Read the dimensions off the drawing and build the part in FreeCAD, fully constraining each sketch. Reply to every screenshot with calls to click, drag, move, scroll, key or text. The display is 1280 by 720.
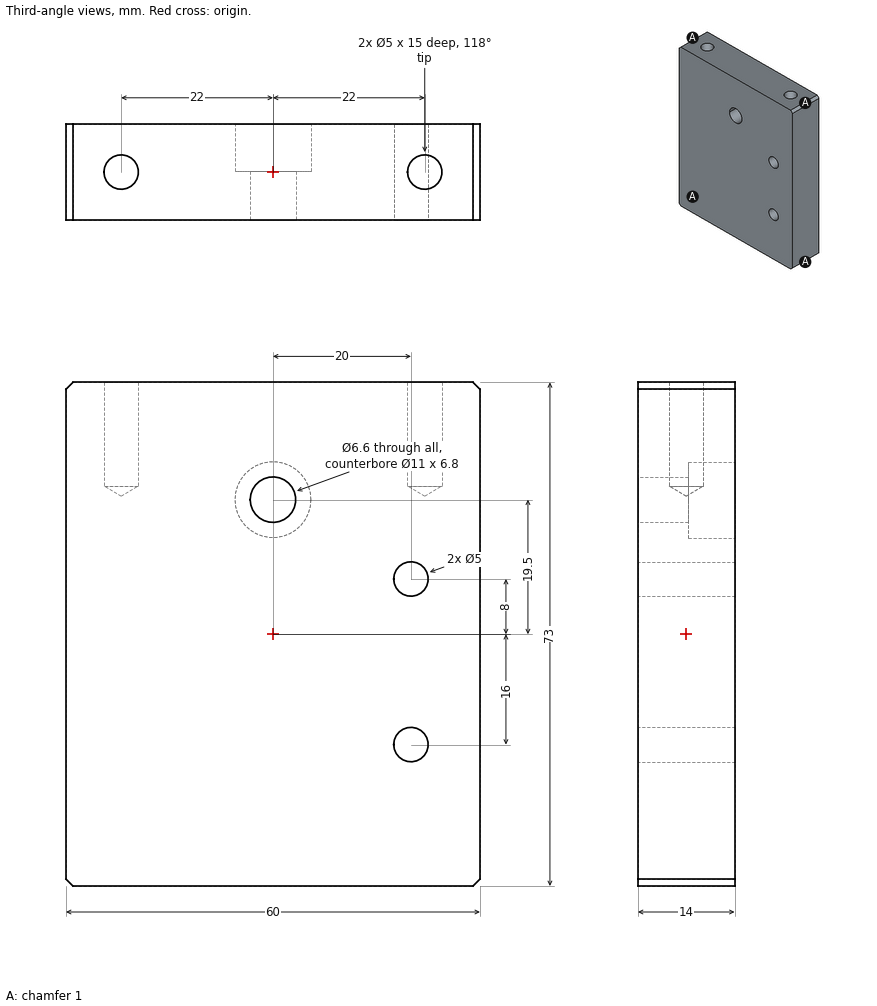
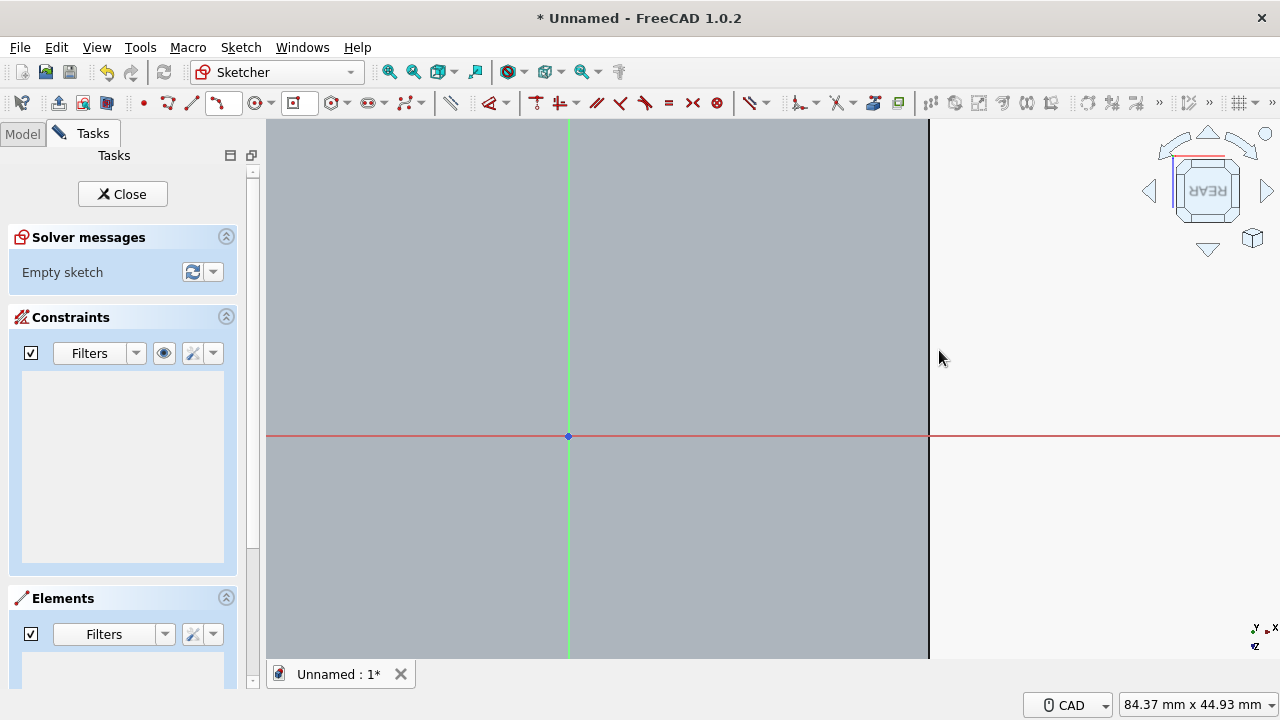
click(256, 104)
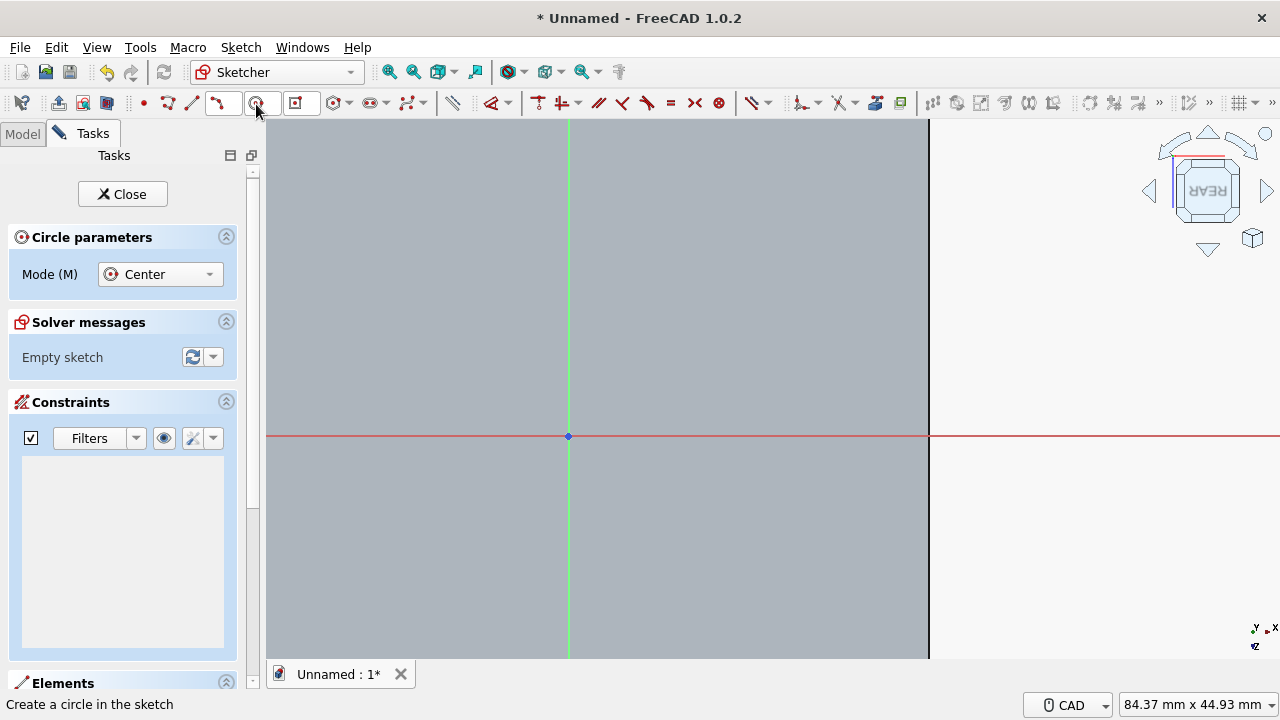
click(809, 532)
click(830, 511)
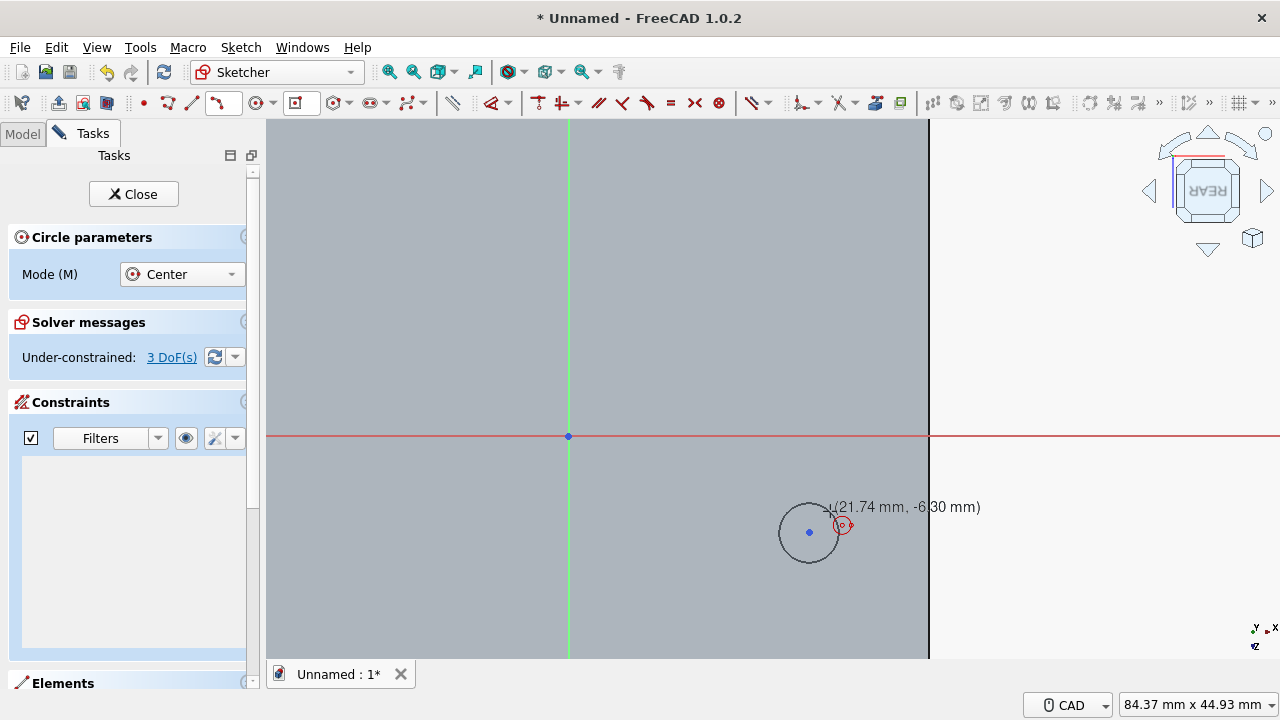
click(809, 244)
click(830, 223)
key(Escape)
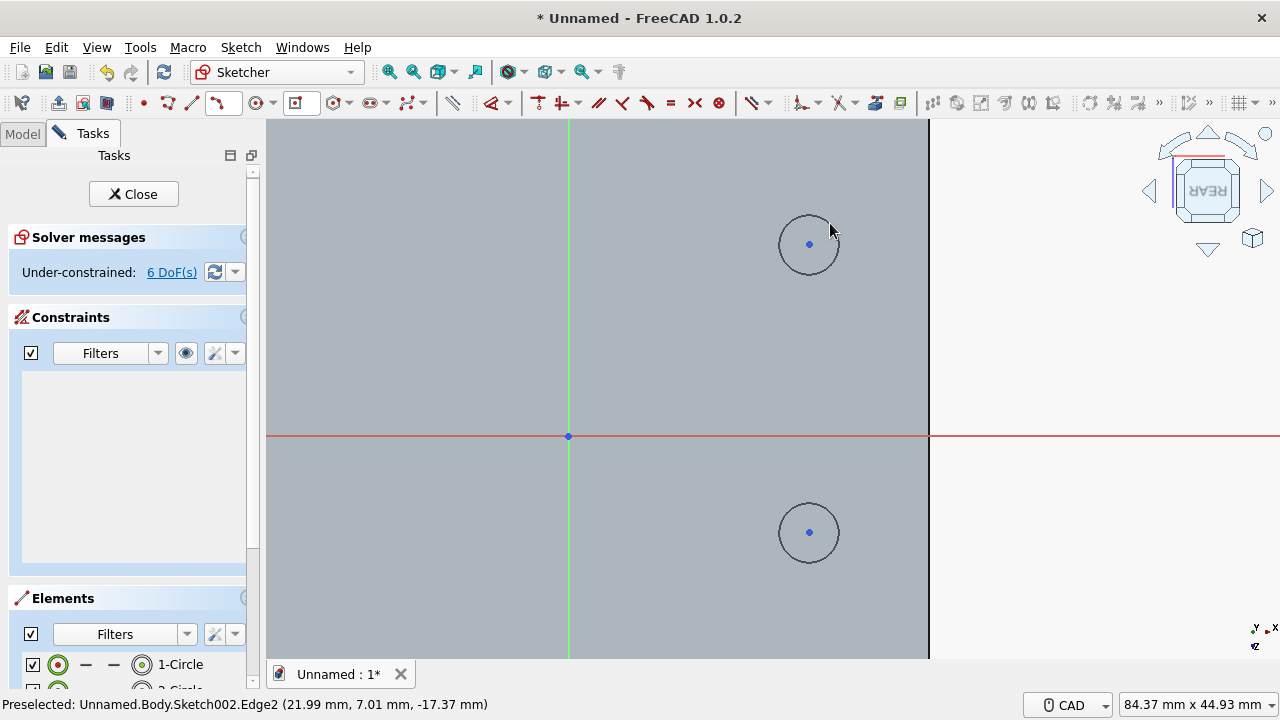
click(830, 512)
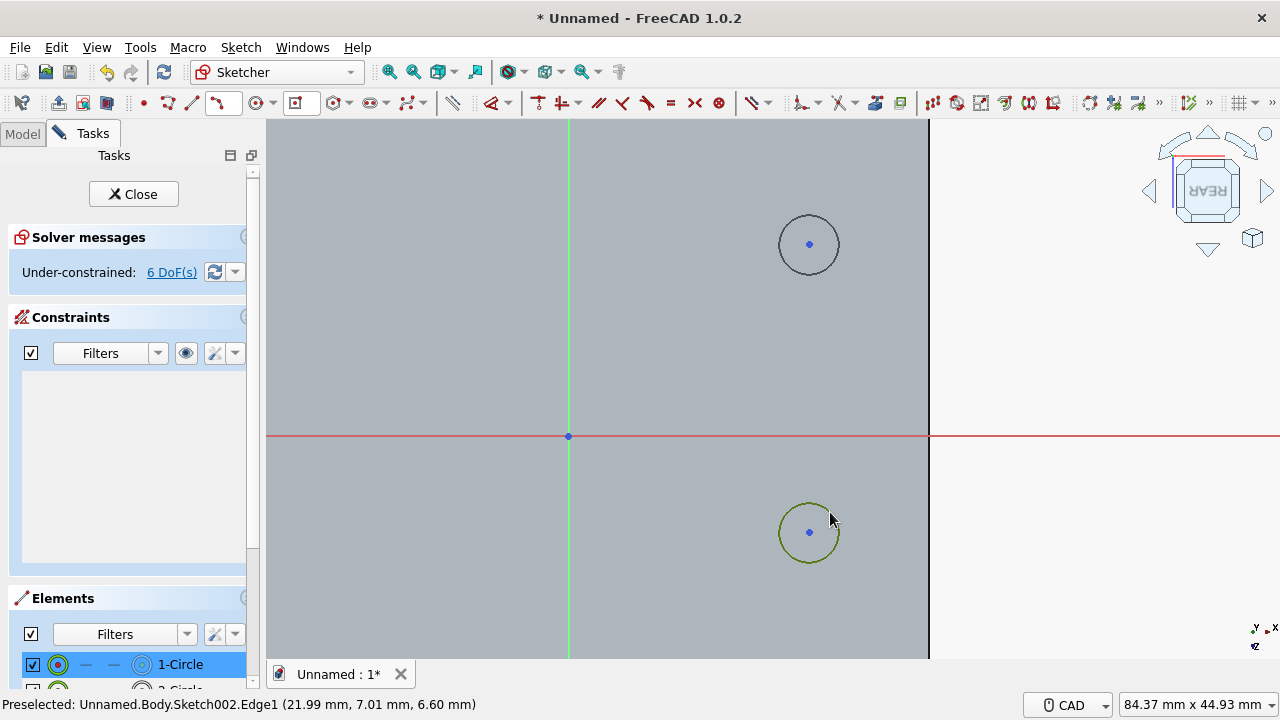
click(830, 224)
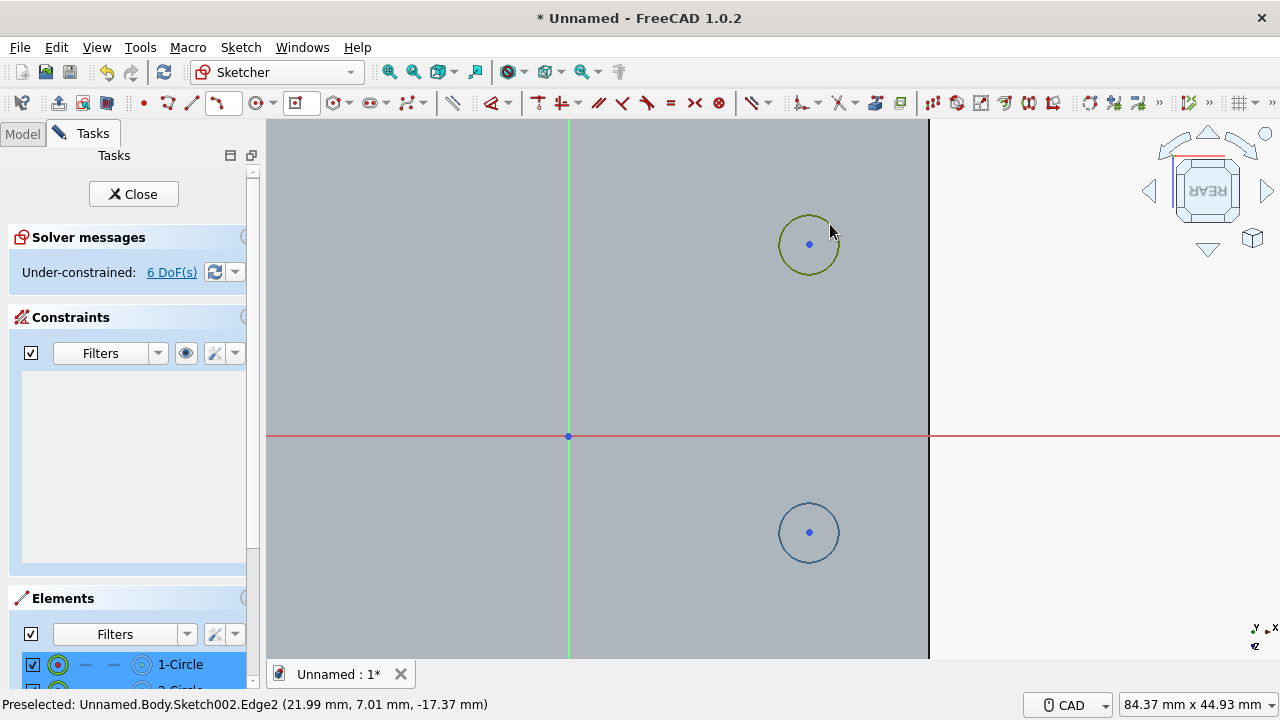
click(672, 104)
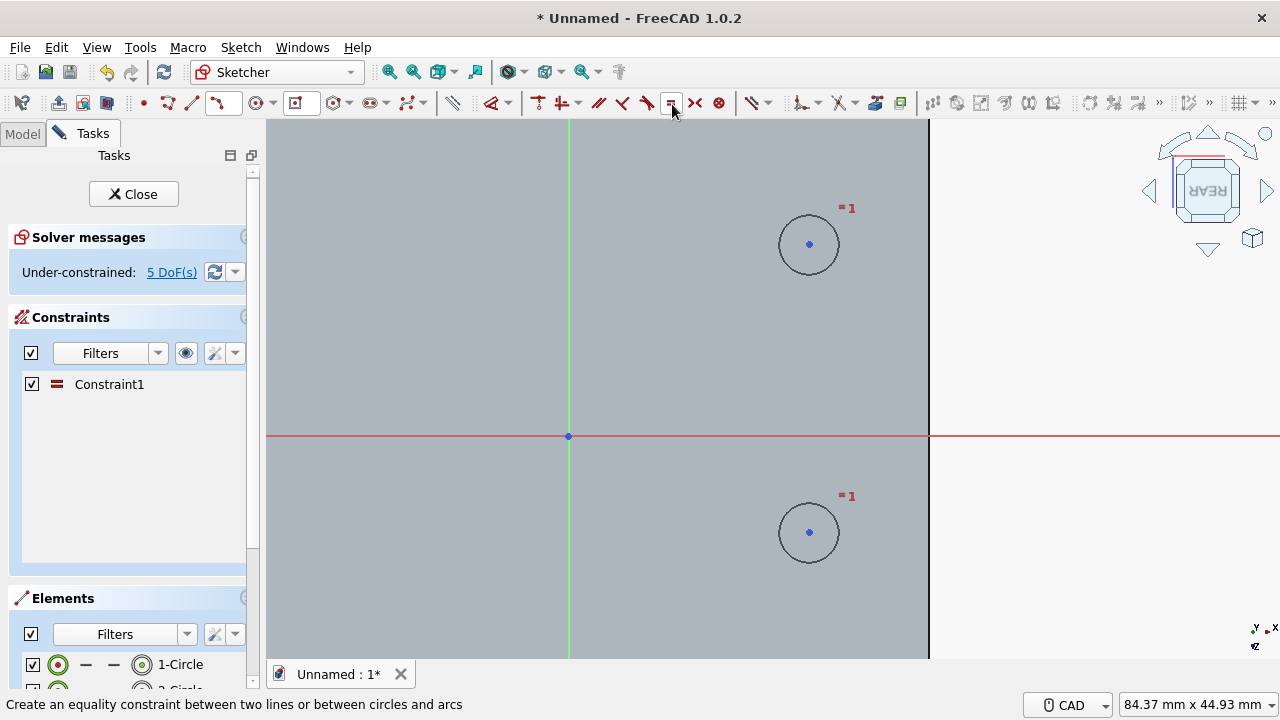
click(809, 533)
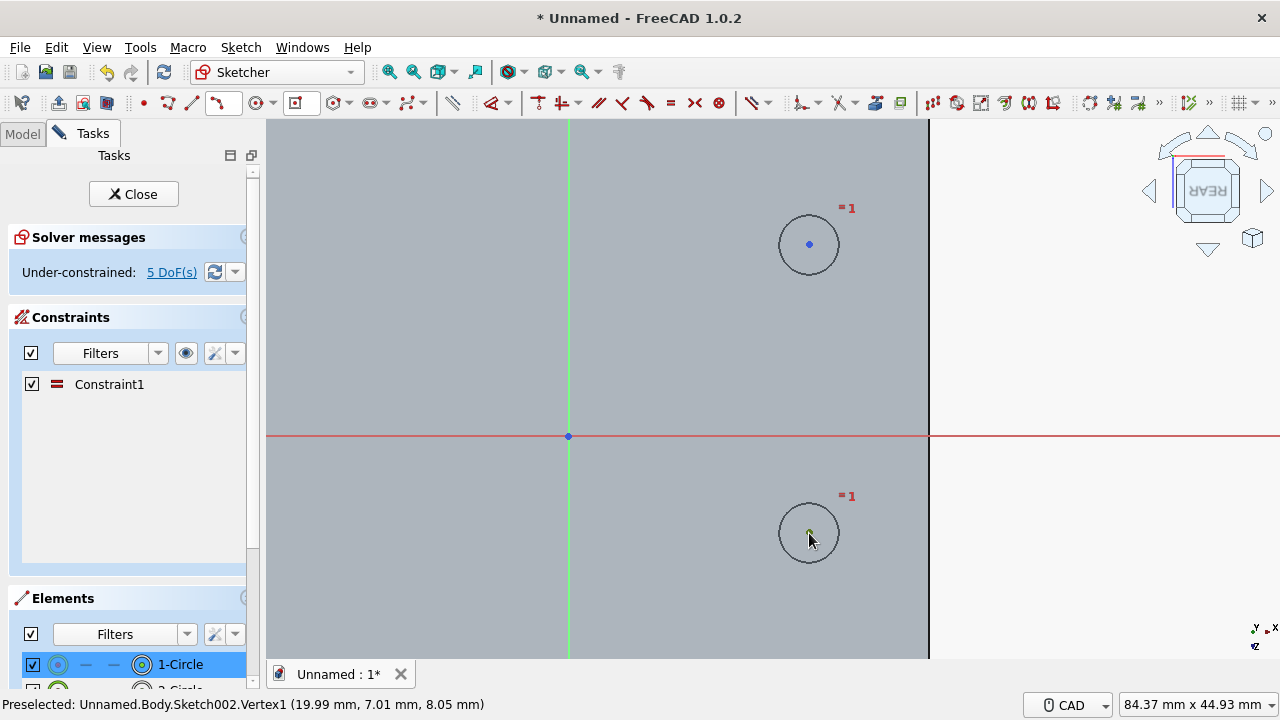
click(809, 245)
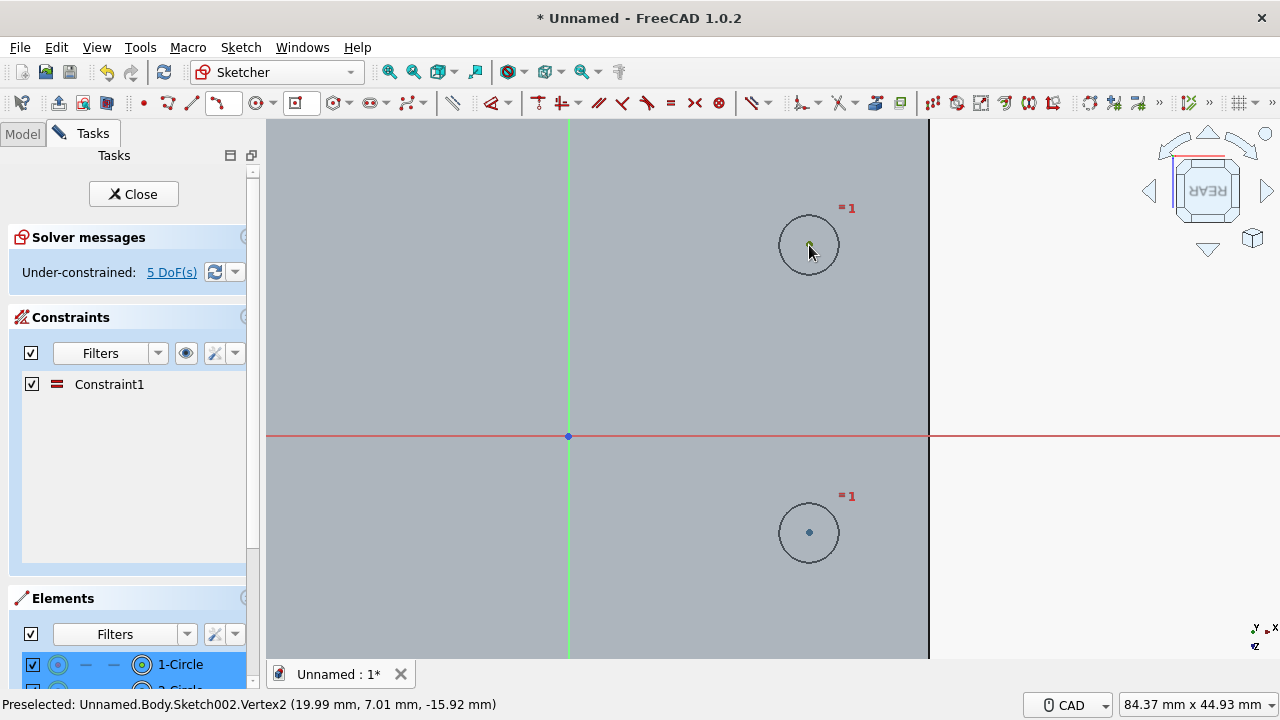
click(580, 104)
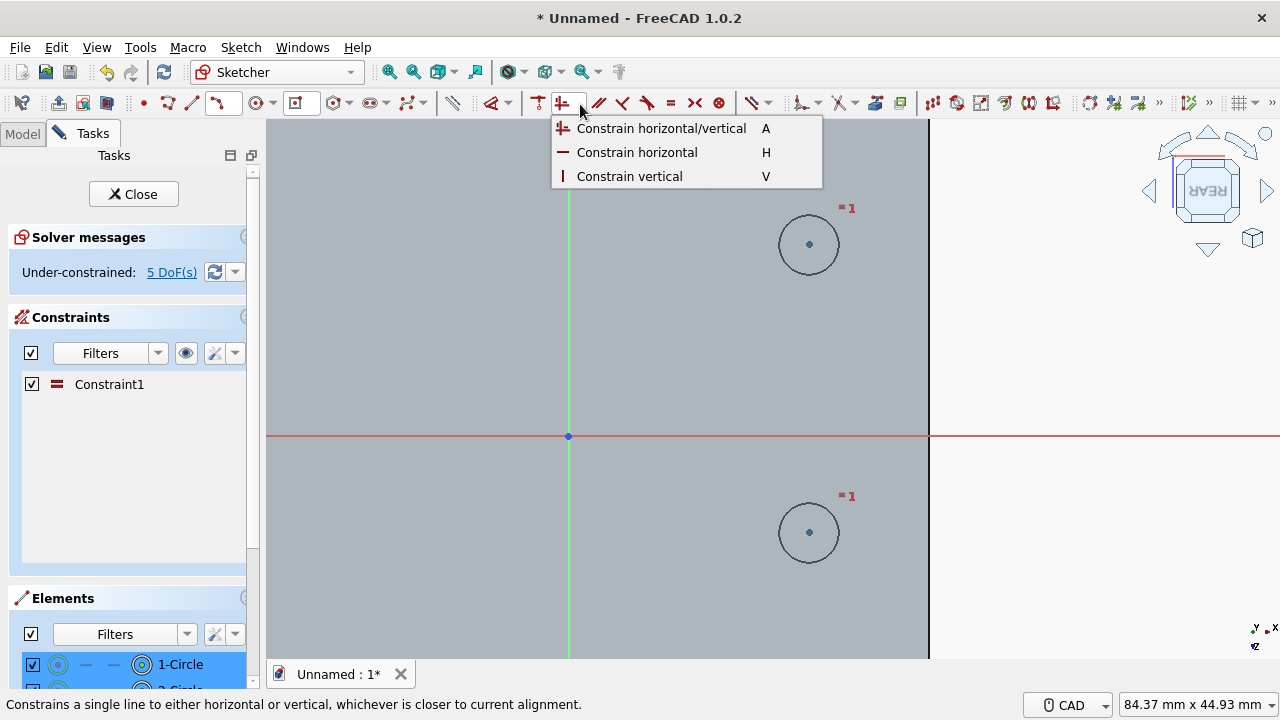
click(687, 176)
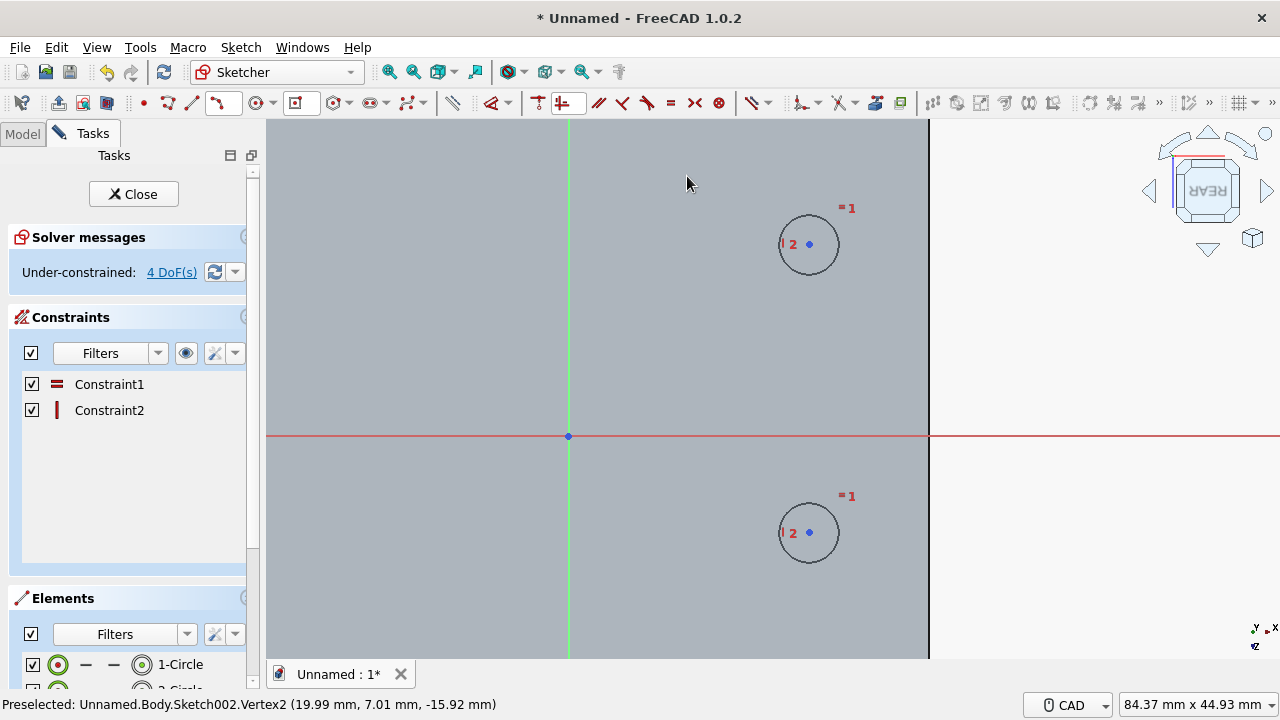
click(492, 104)